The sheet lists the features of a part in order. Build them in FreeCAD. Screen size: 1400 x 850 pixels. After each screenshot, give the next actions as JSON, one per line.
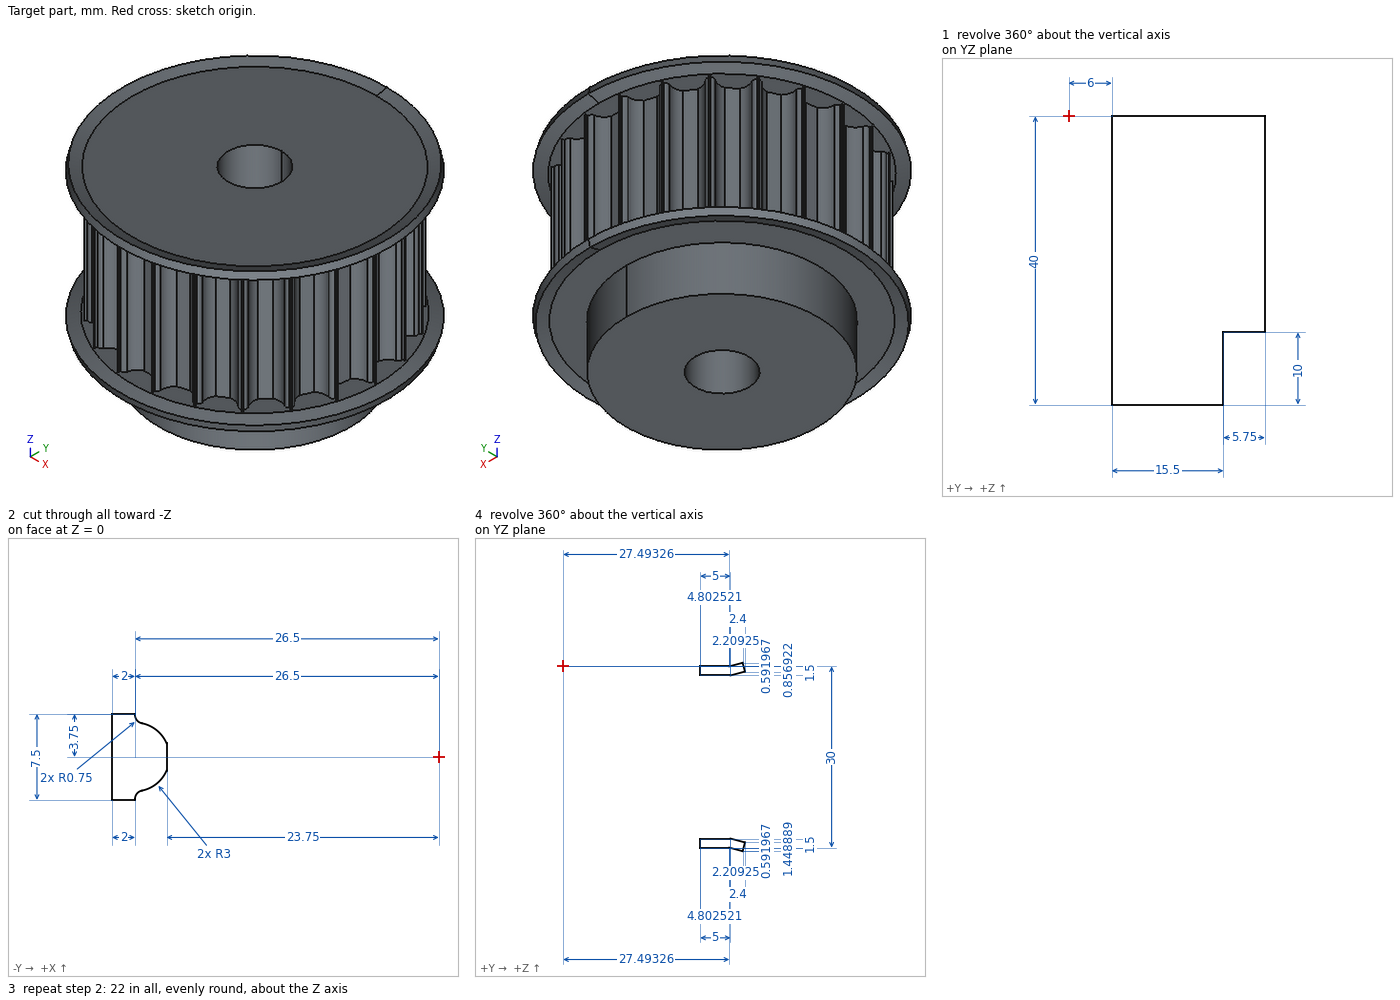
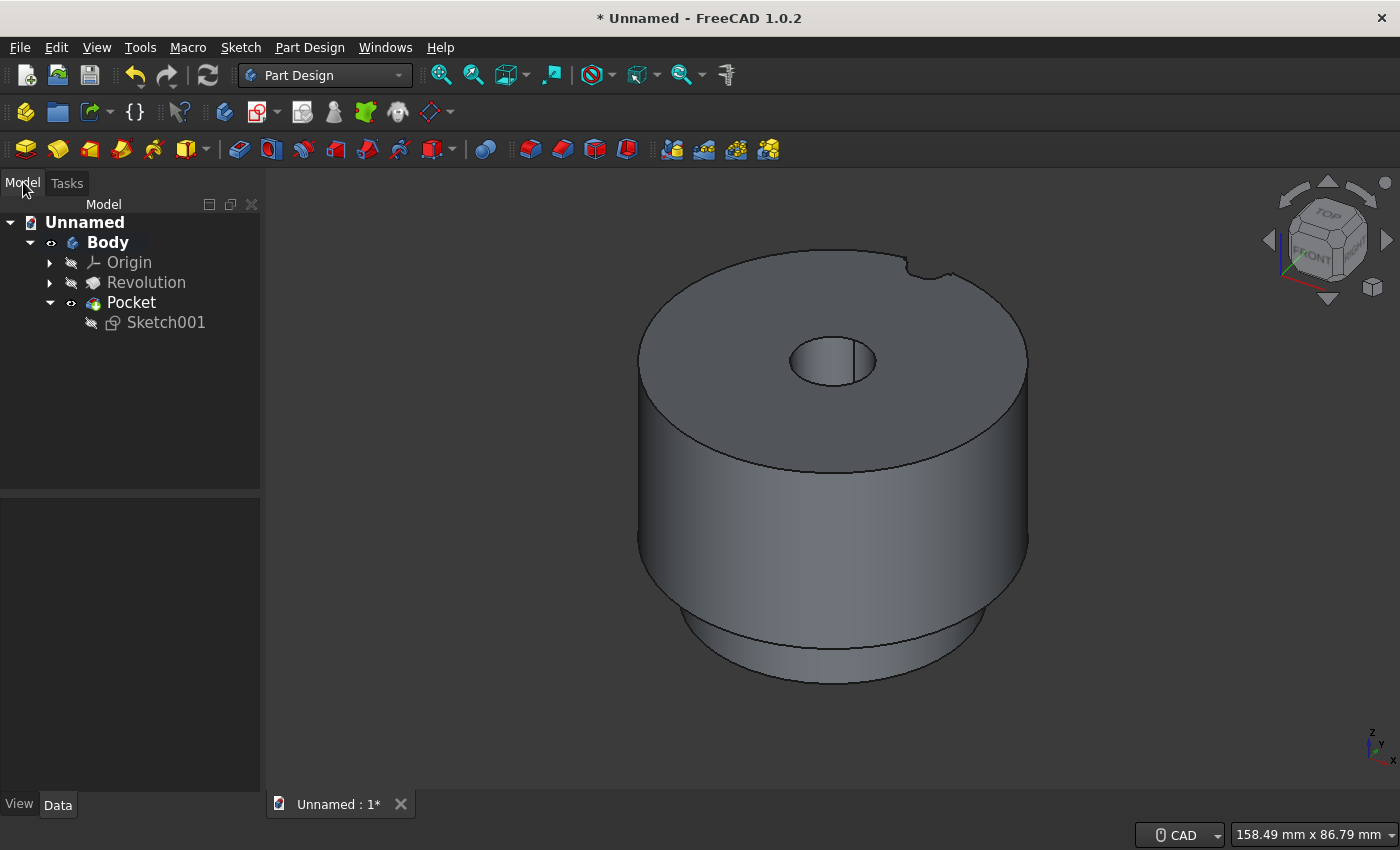
{"action": "left_click", "coordinate": [116, 303]}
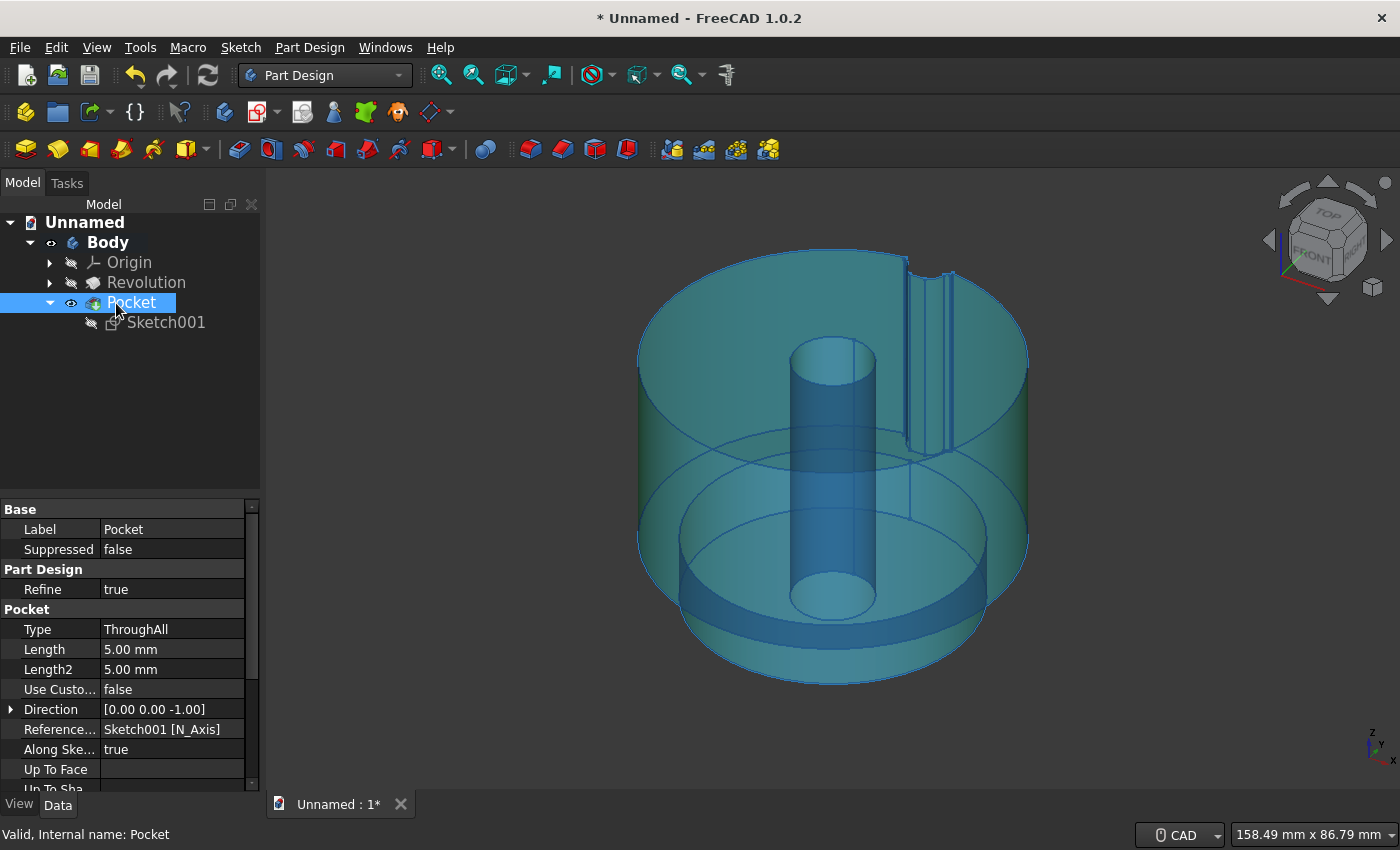
{"action": "left_click", "coordinate": [736, 150]}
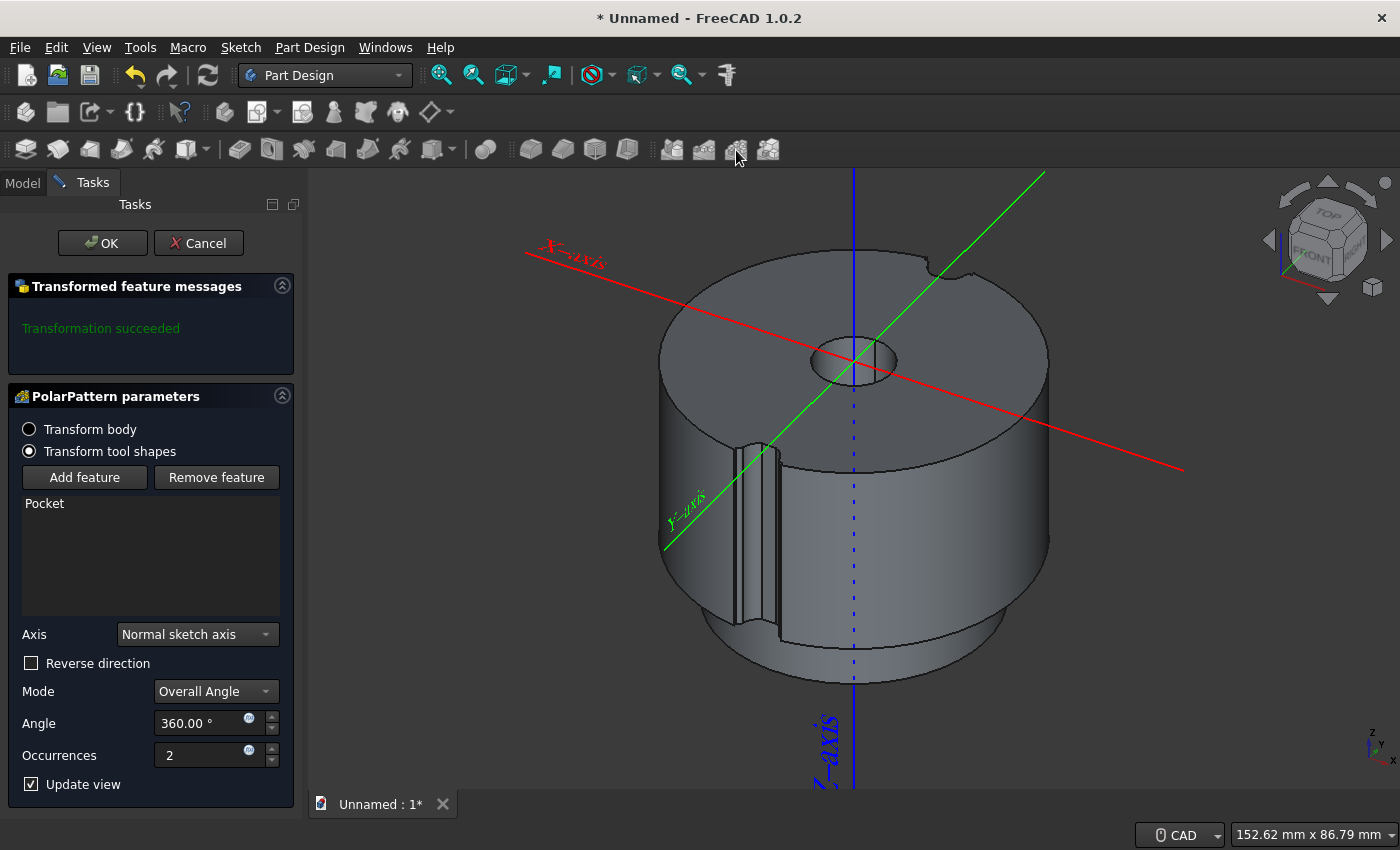
{"action": "left_click", "coordinate": [198, 634]}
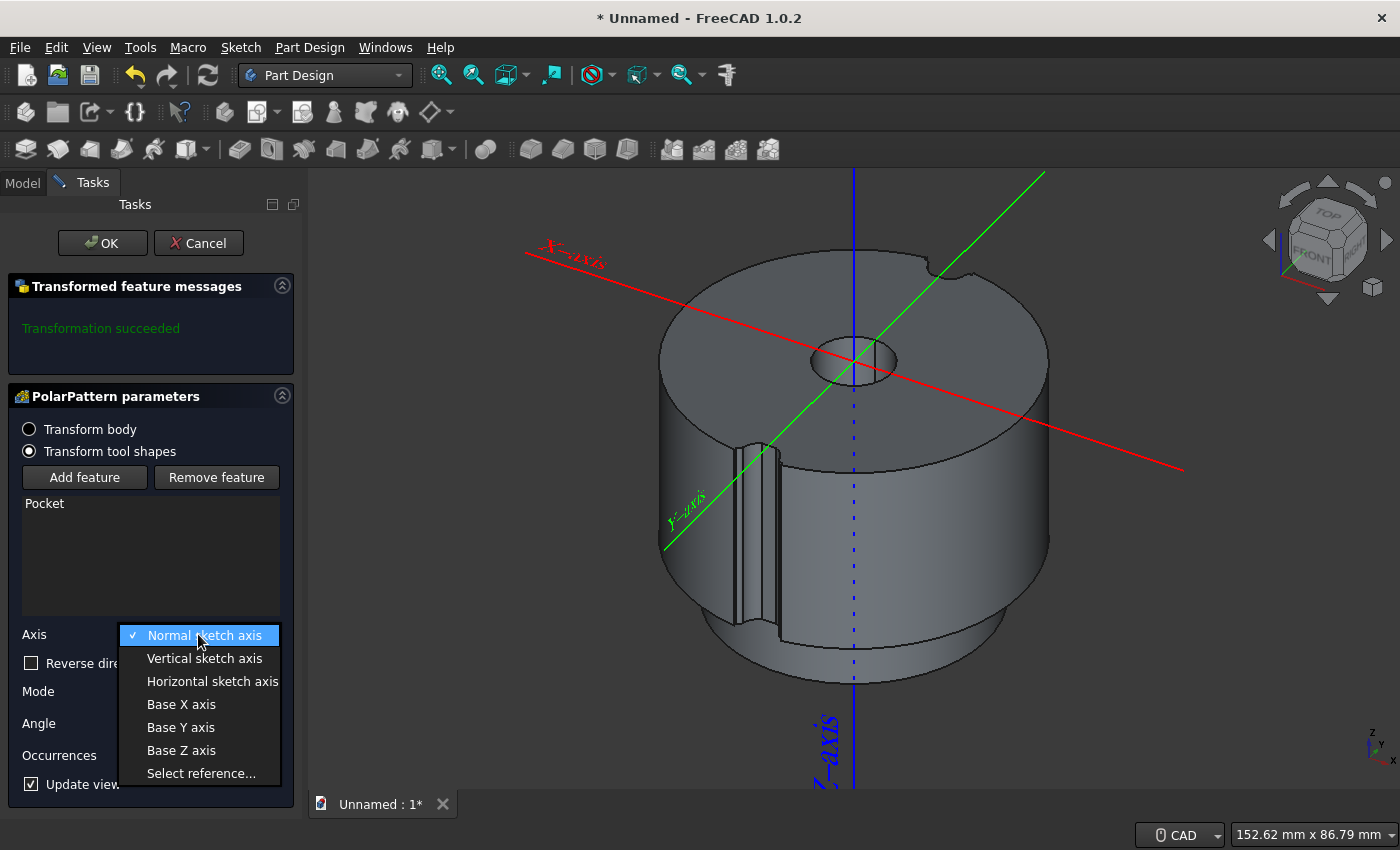
{"action": "left_click", "coordinate": [198, 750]}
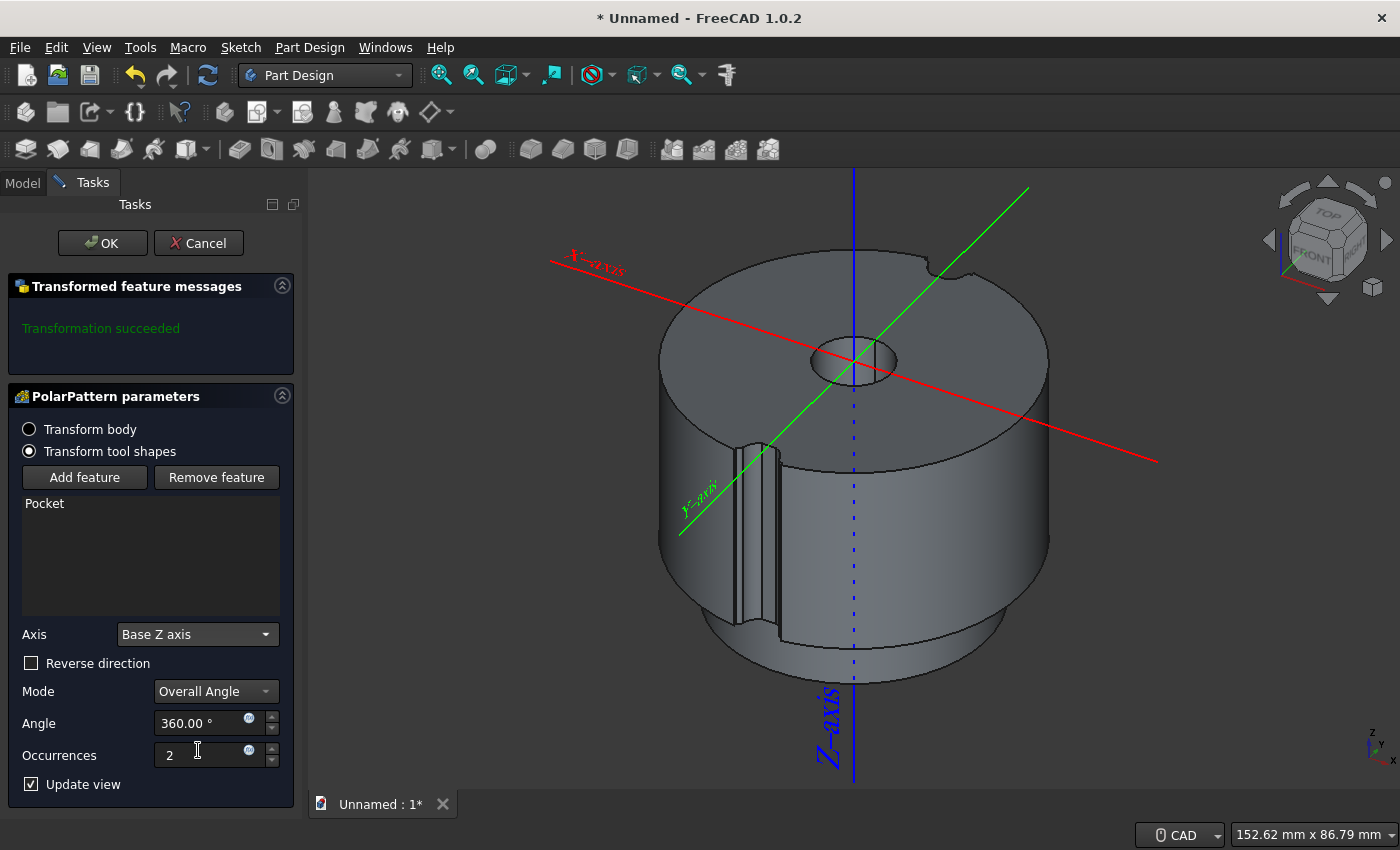
{"action": "triple_click", "coordinate": [209, 755]}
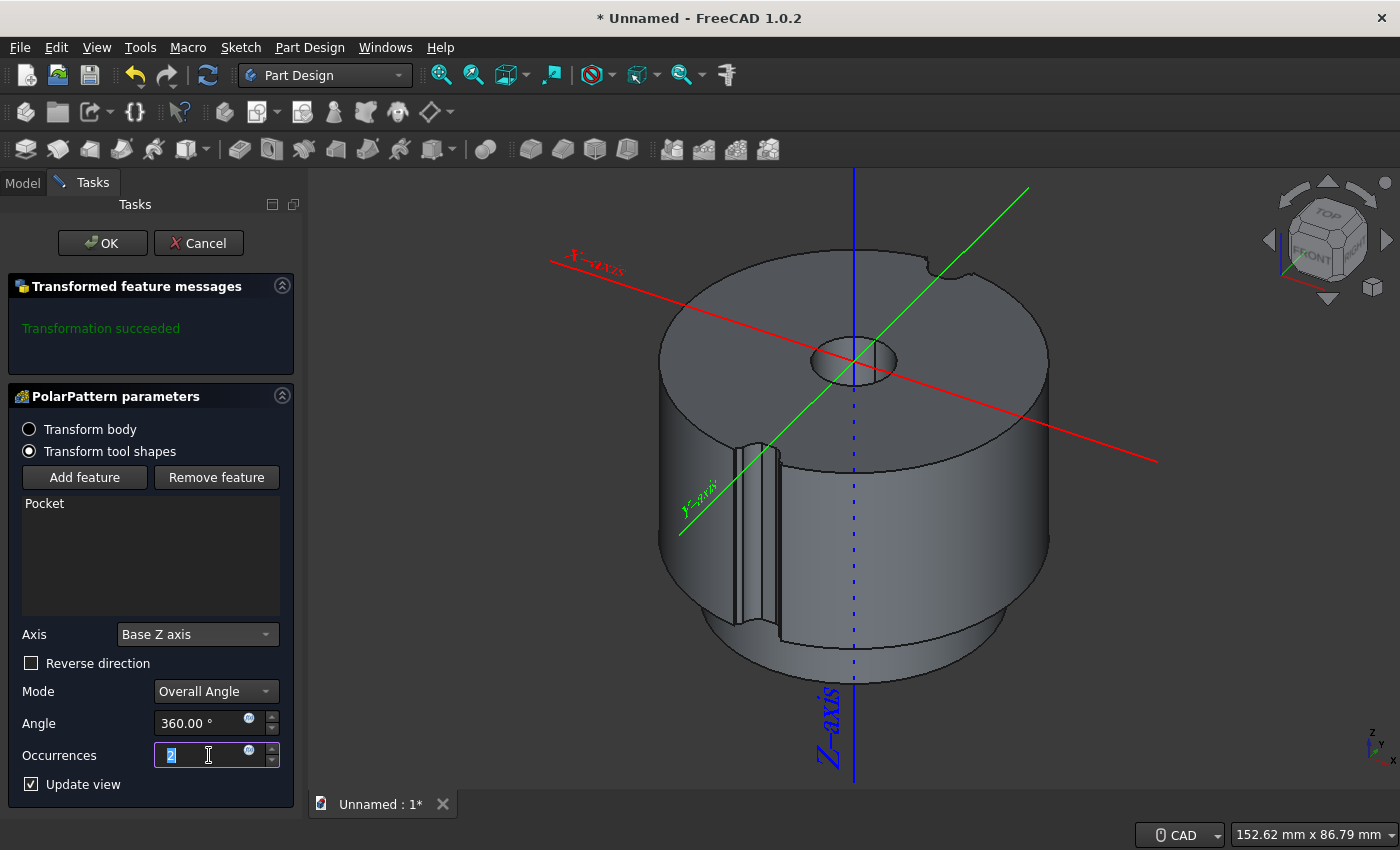
{"action": "type", "text": "22"}
{"action": "key", "text": "Tab"}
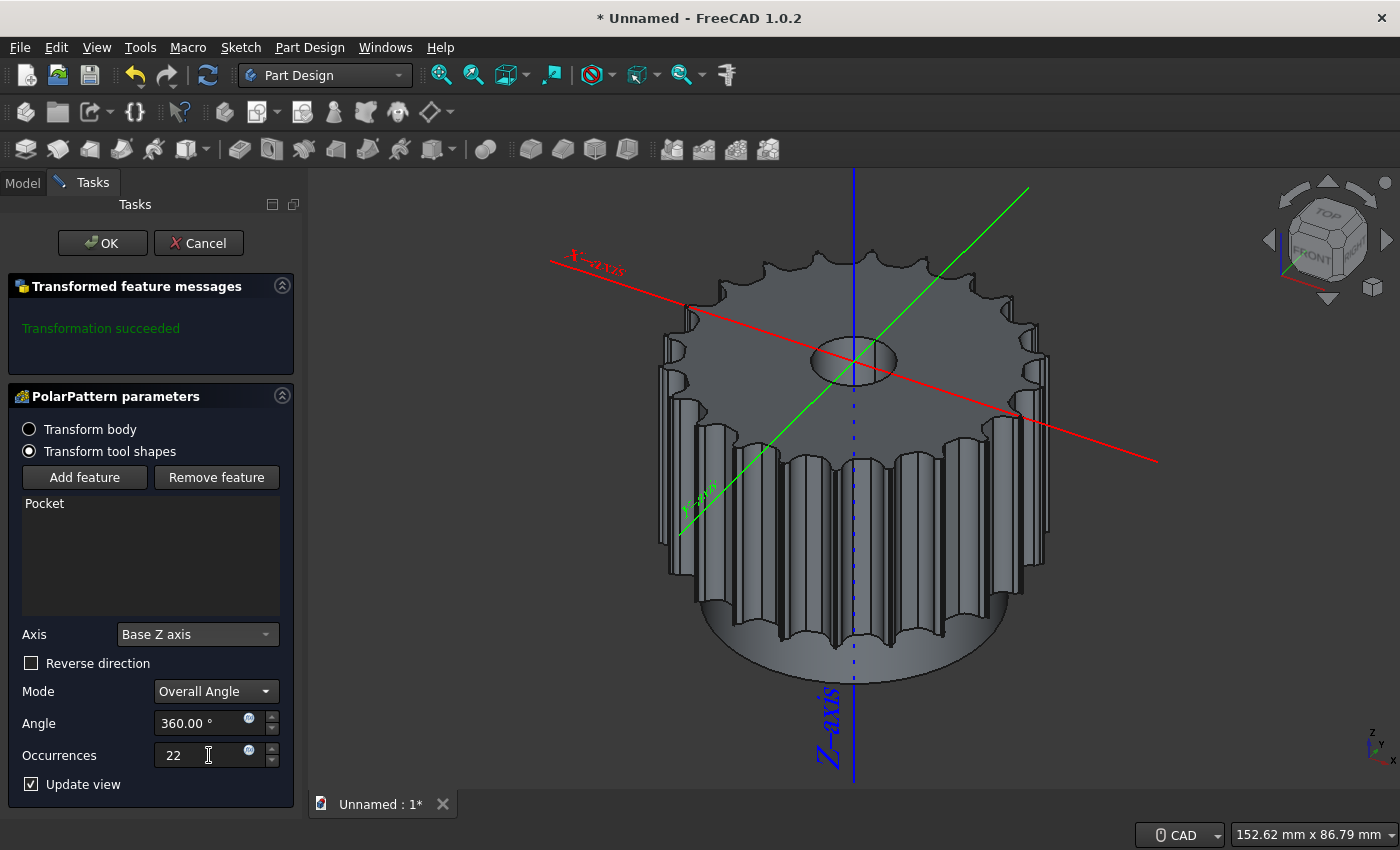
{"action": "left_click", "coordinate": [103, 243]}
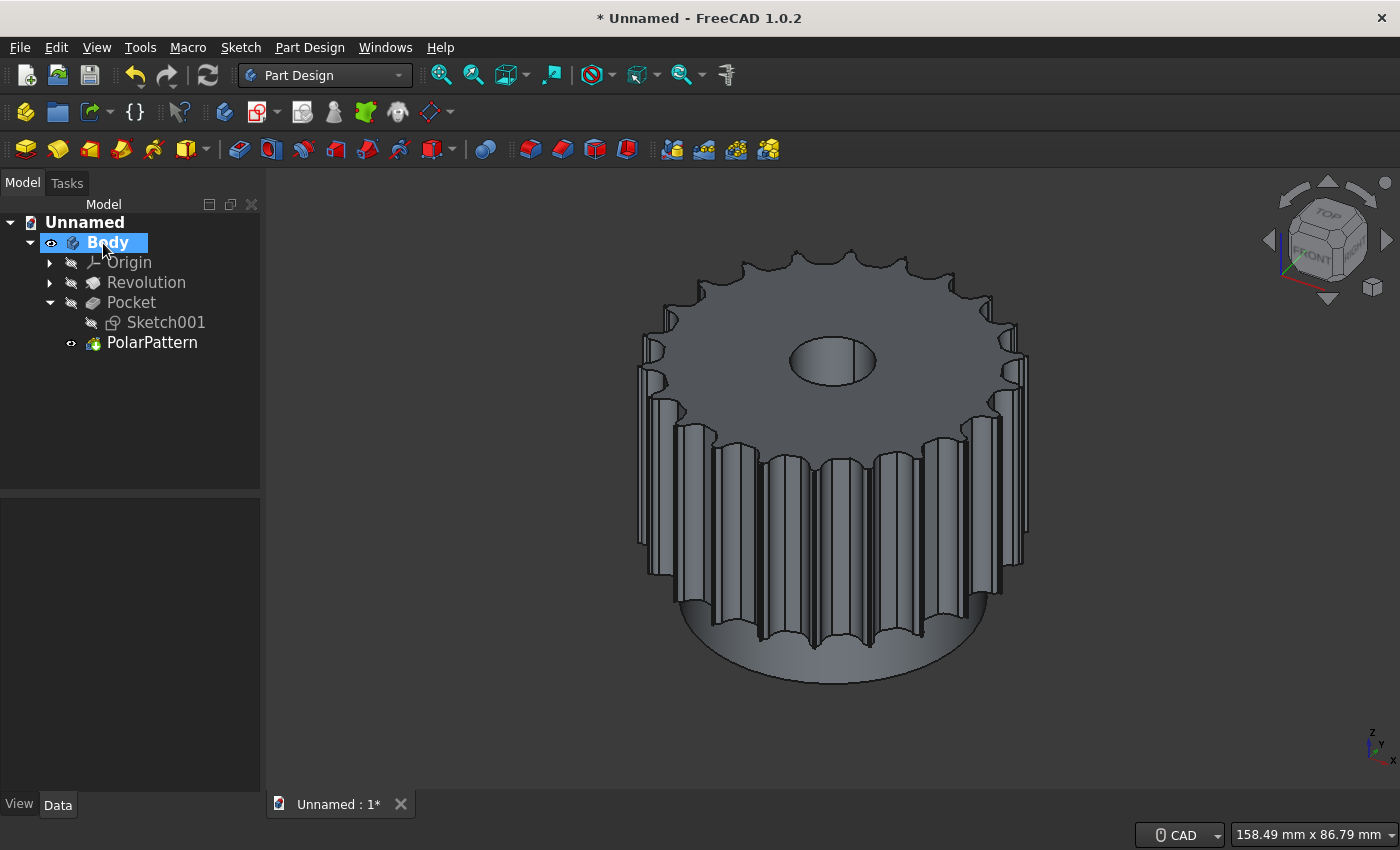
{"action": "left_click", "coordinate": [258, 112]}